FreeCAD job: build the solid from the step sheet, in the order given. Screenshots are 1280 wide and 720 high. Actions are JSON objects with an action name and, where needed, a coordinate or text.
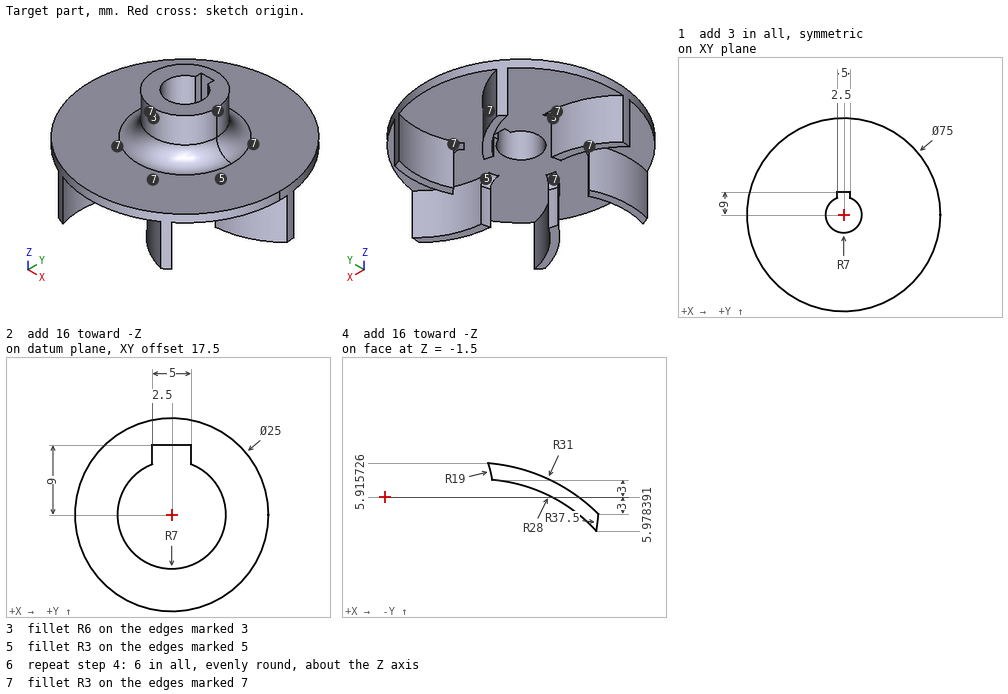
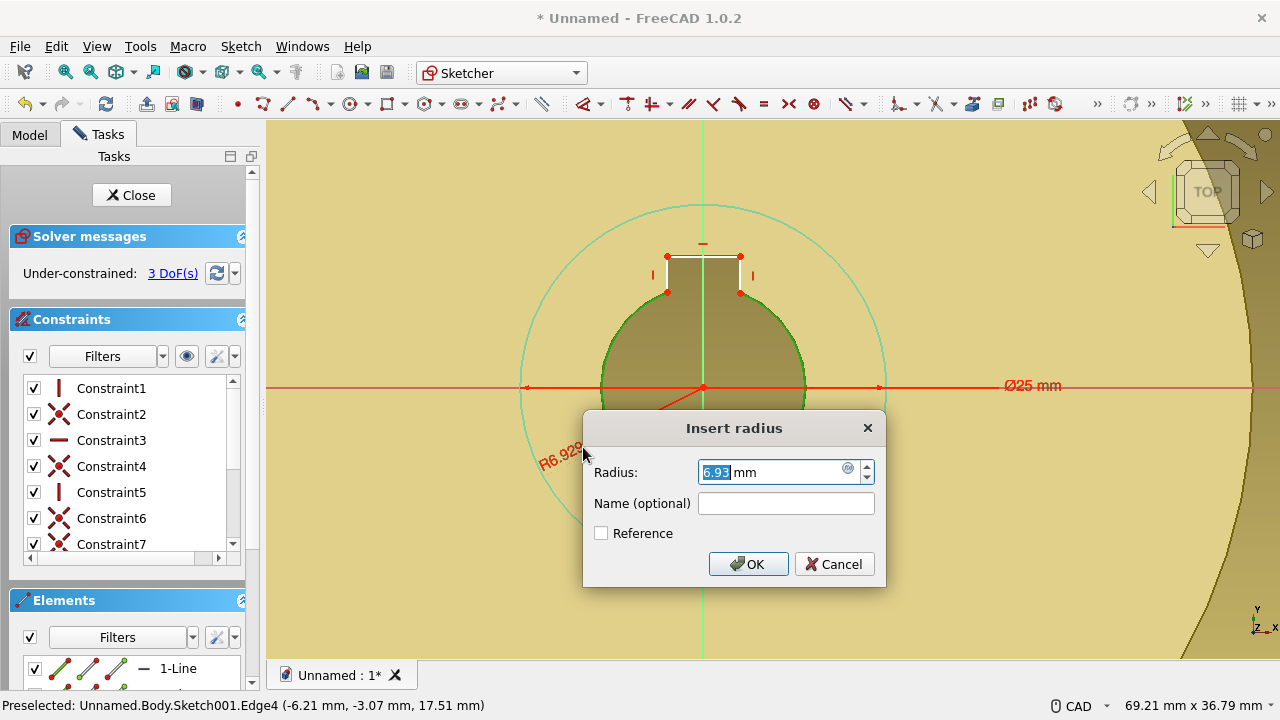
{"action": "type", "text": "7"}
{"action": "key", "text": "Return"}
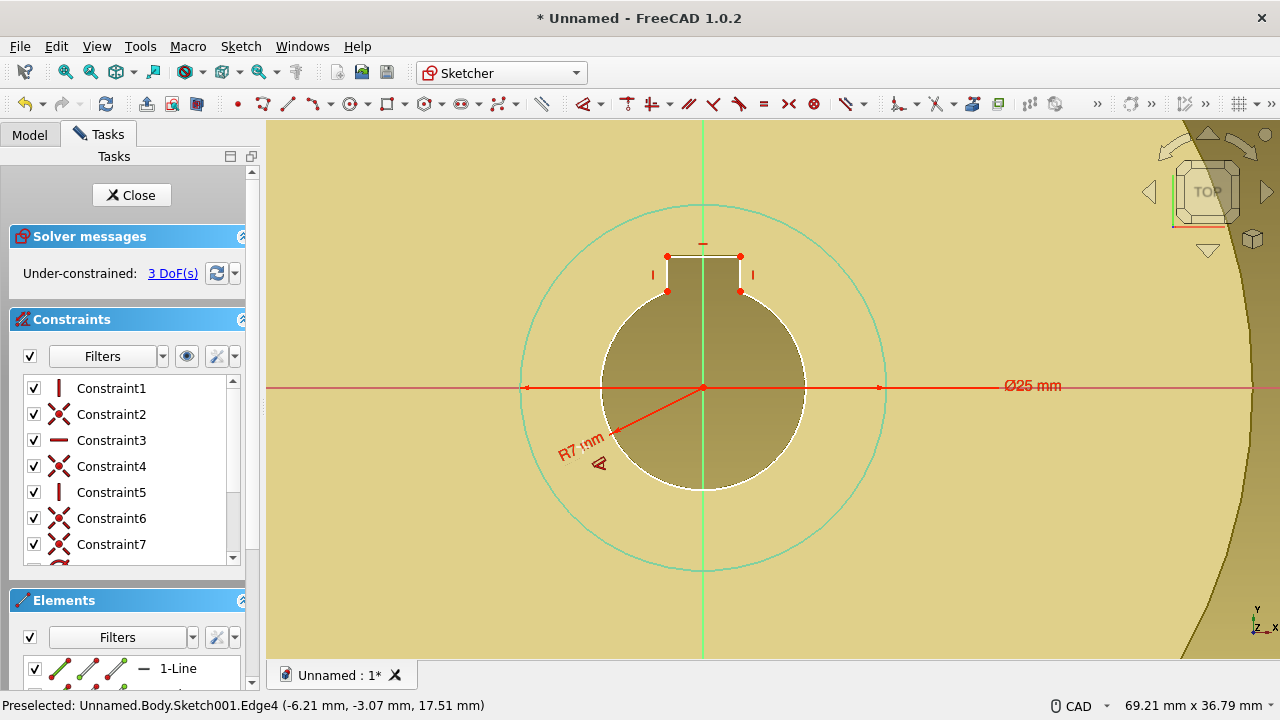
{"action": "left_click", "coordinate": [689, 257]}
{"action": "left_click", "coordinate": [687, 223]}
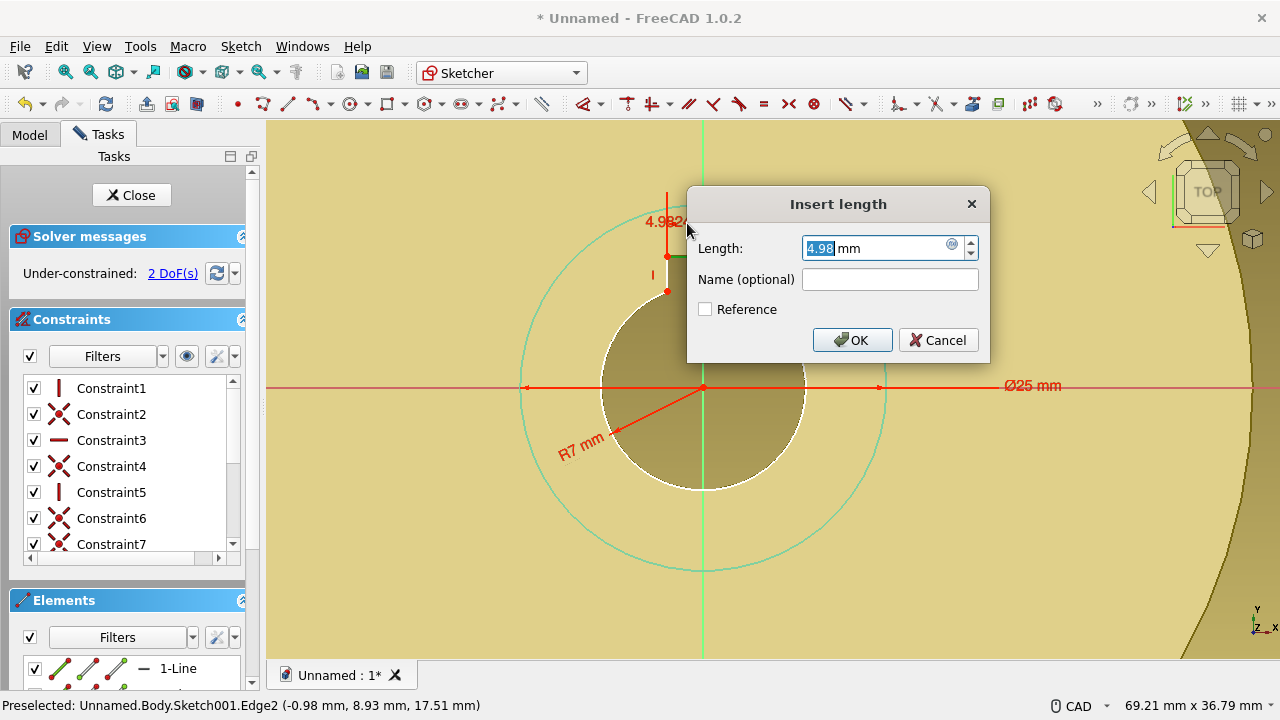
{"action": "type", "text": "5"}
{"action": "key", "text": "Return"}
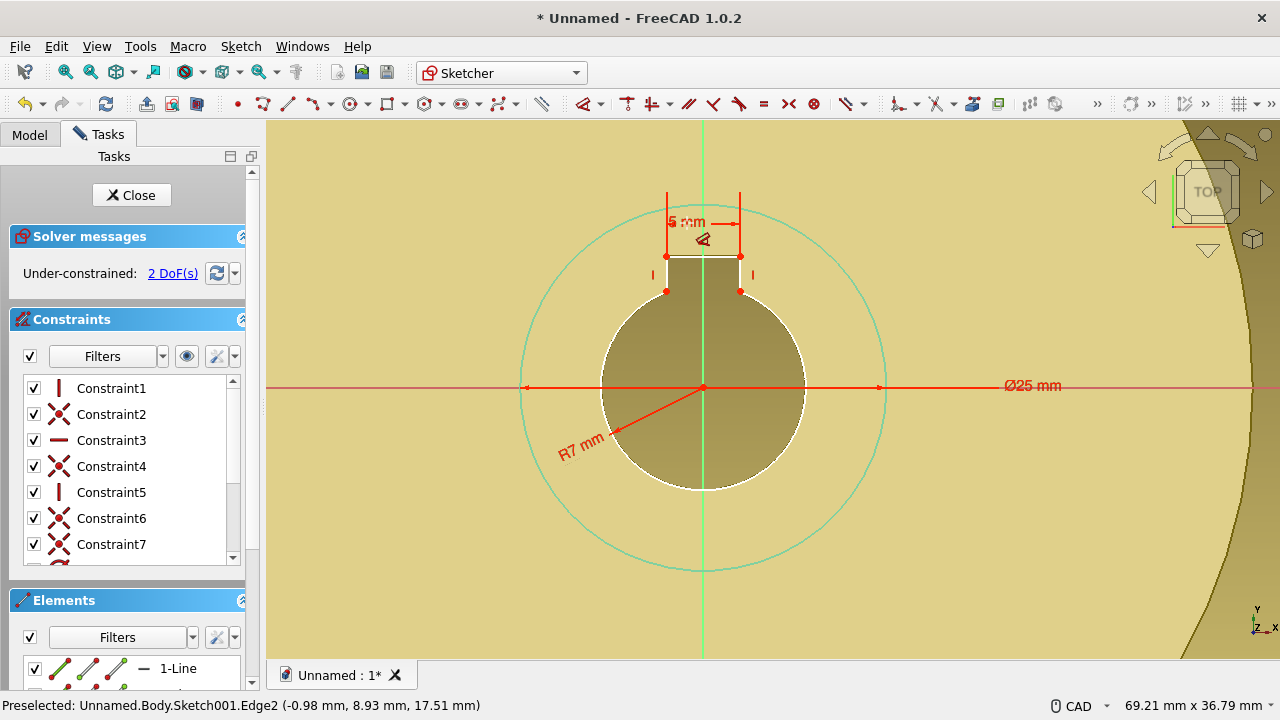
{"action": "left_click", "coordinate": [667, 257]}
{"action": "left_click", "coordinate": [633, 292]}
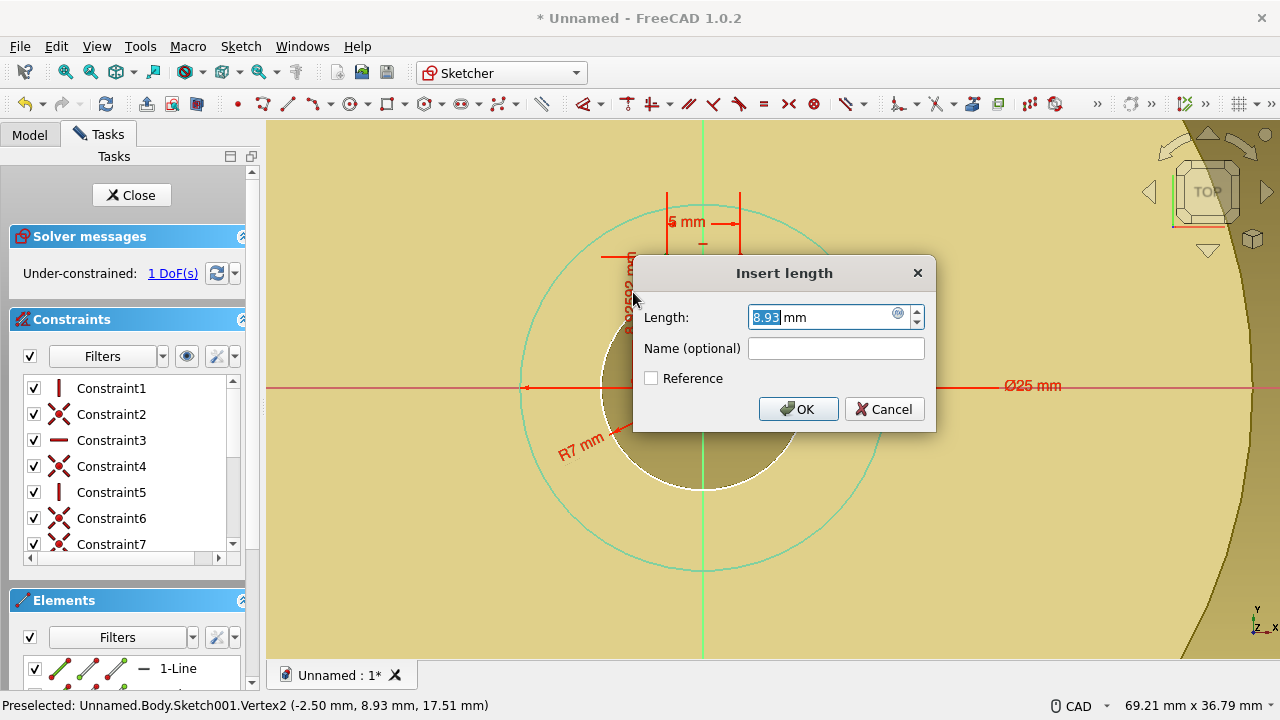
{"action": "type", "text": "9"}
{"action": "key", "text": "Return"}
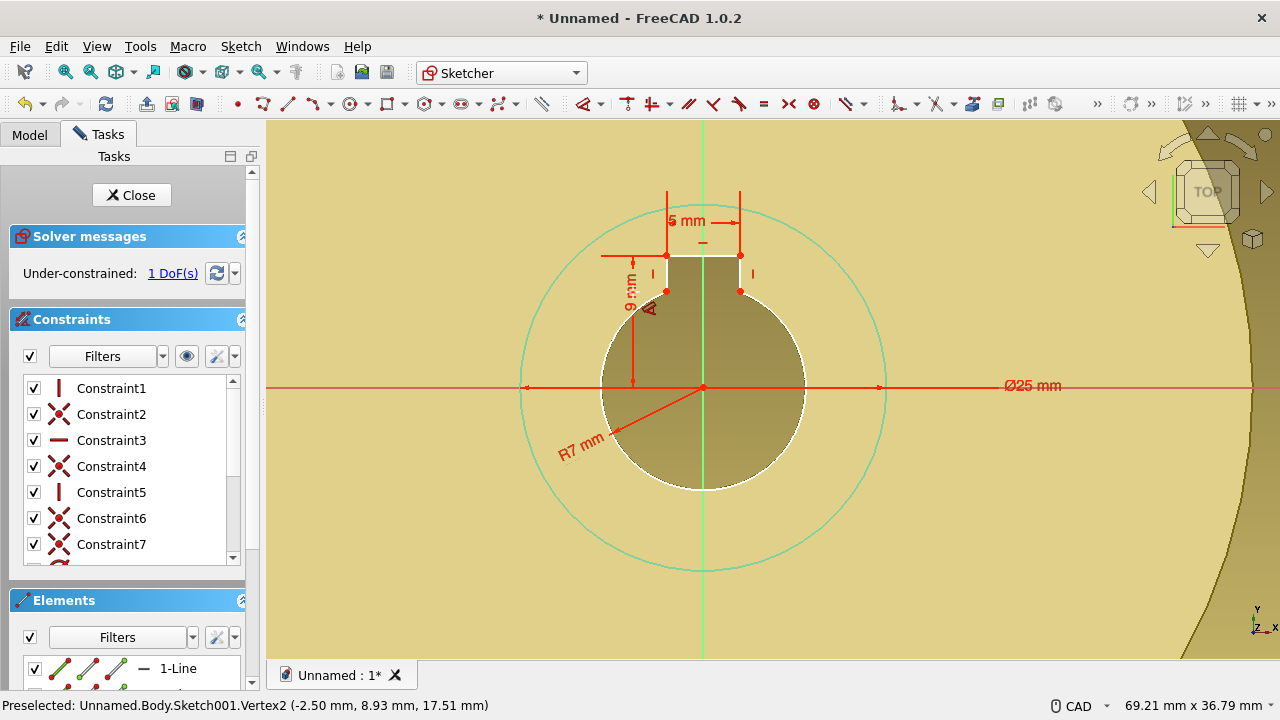
{"action": "left_click", "coordinate": [667, 292]}
{"action": "left_click", "coordinate": [685, 422]}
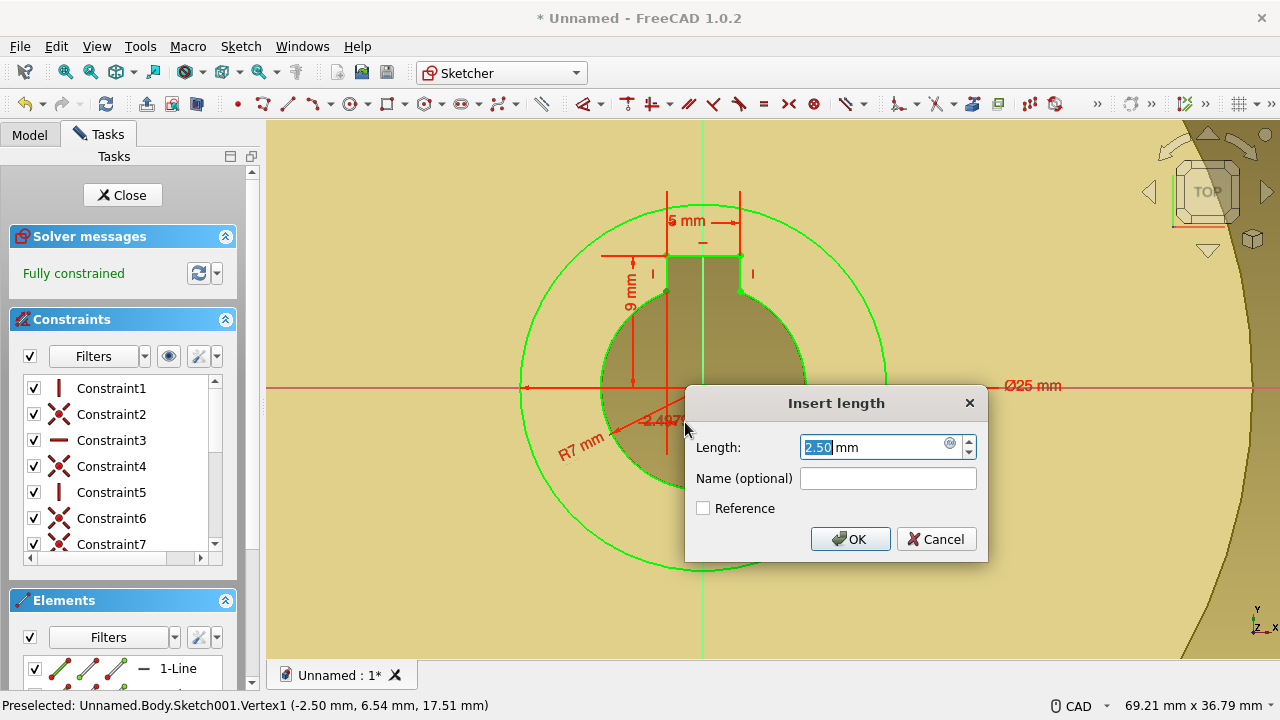
{"action": "type", "text": "2.5"}
{"action": "key", "text": "Return"}
{"action": "key", "text": "Escape"}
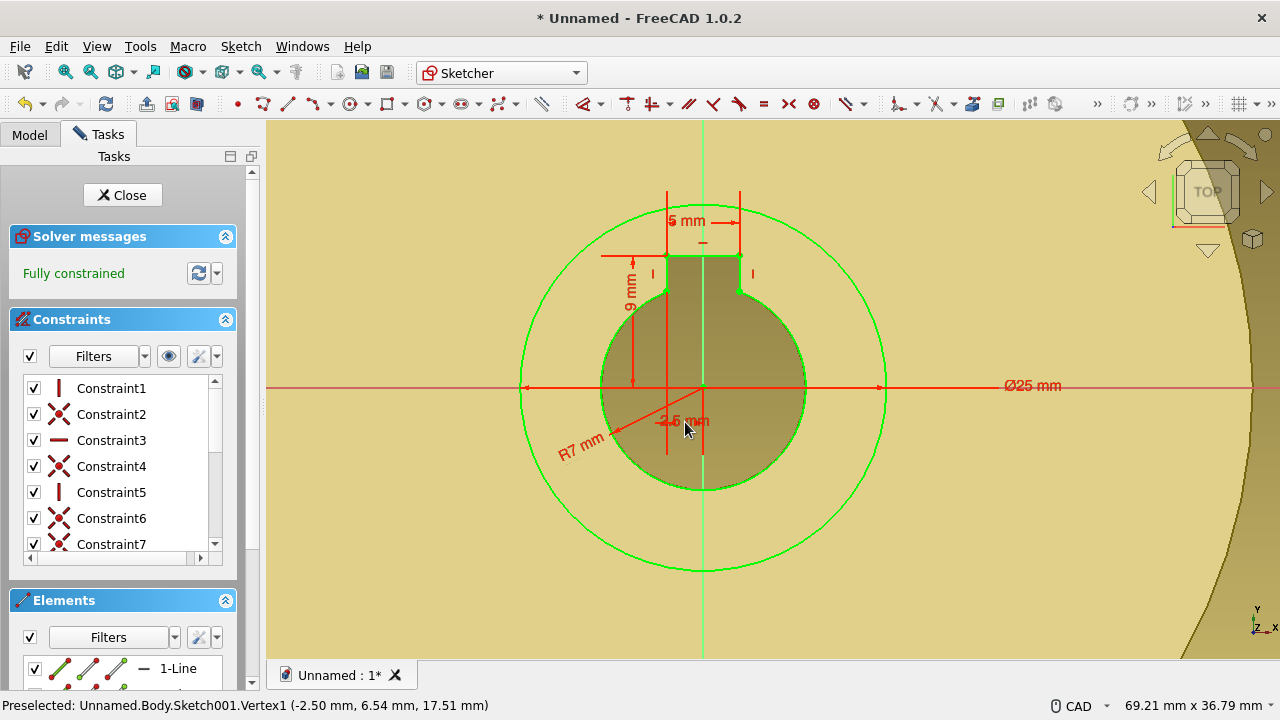
{"action": "left_click", "coordinate": [123, 195]}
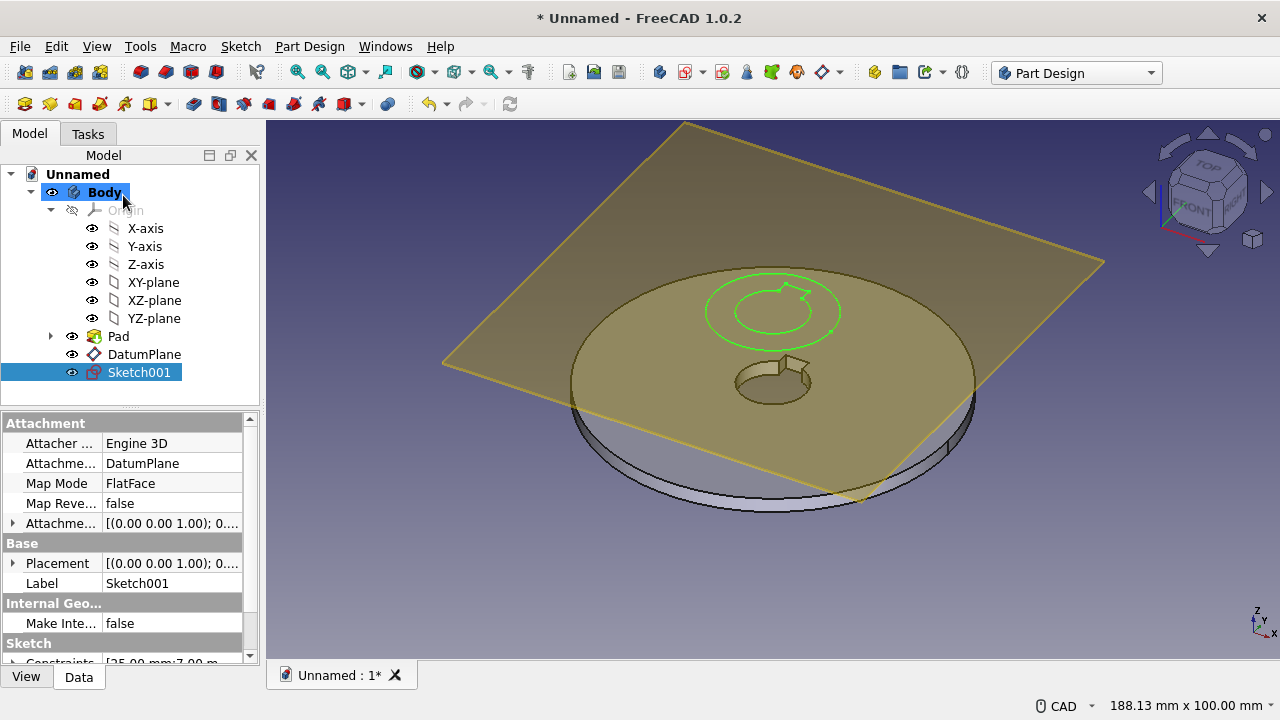
{"action": "left_click", "coordinate": [25, 104]}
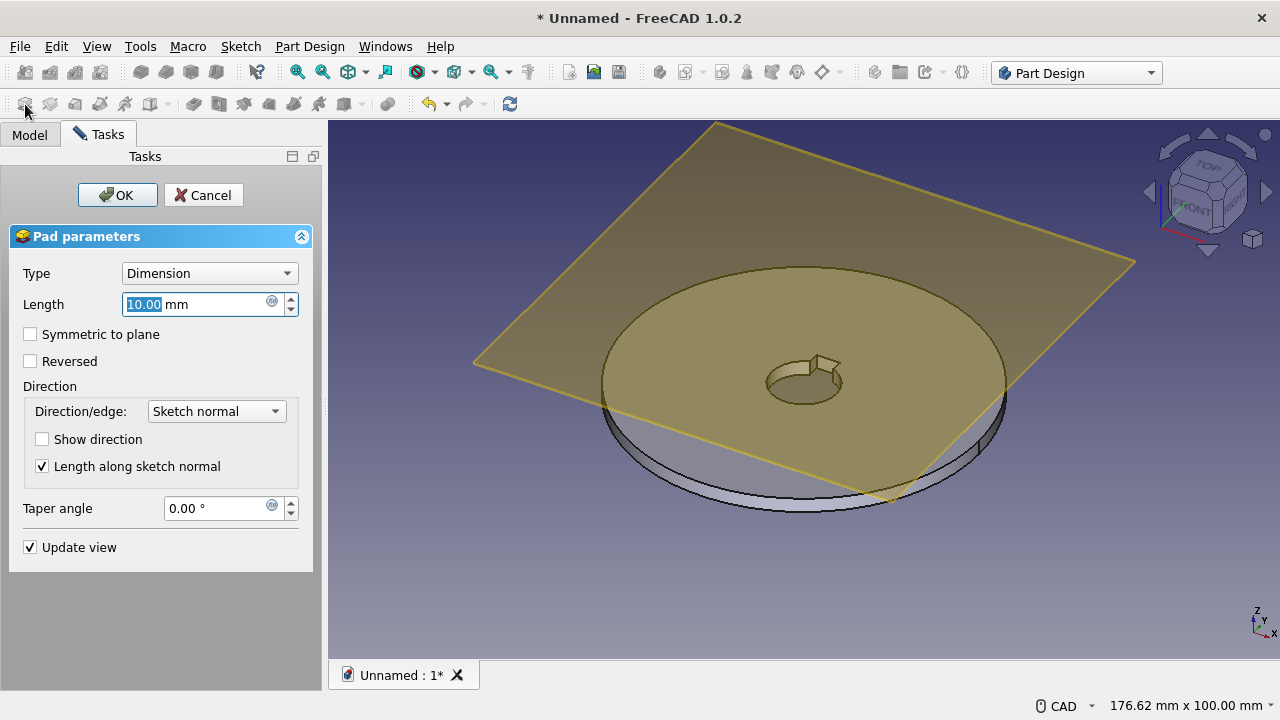
{"action": "type", "text": "16"}
{"action": "key", "text": "Tab"}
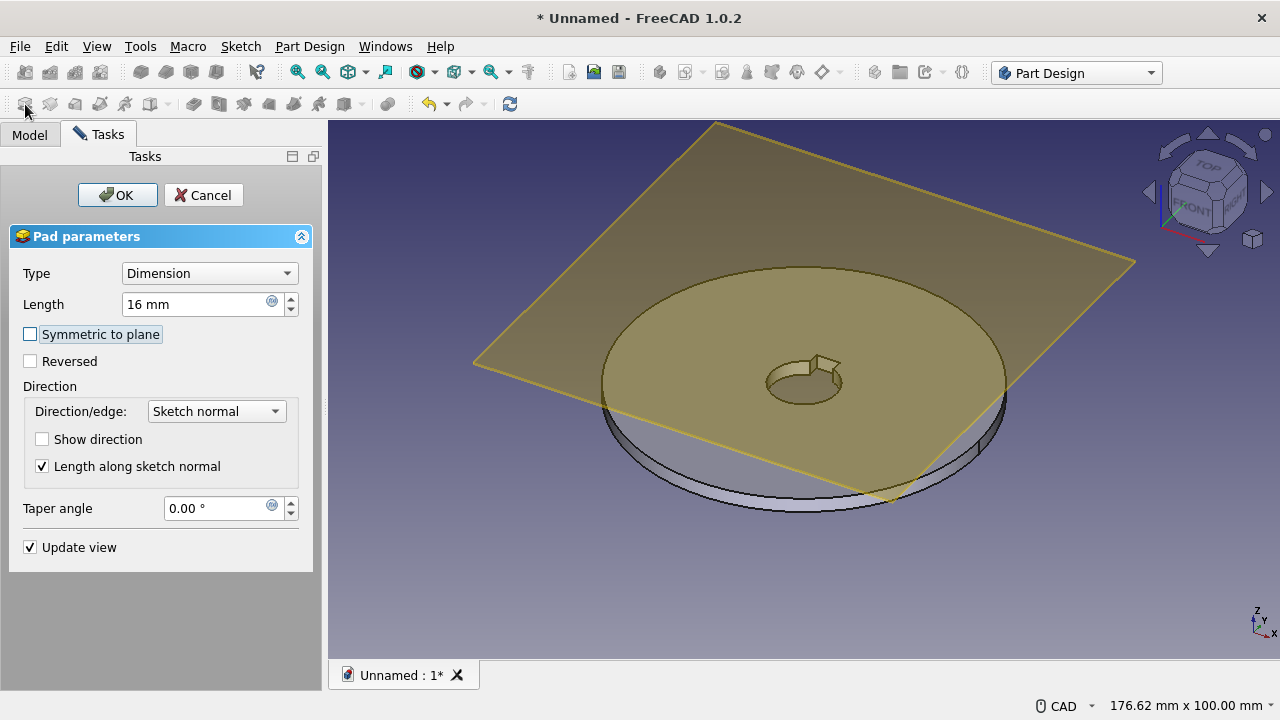
{"action": "left_click", "coordinate": [31, 361]}